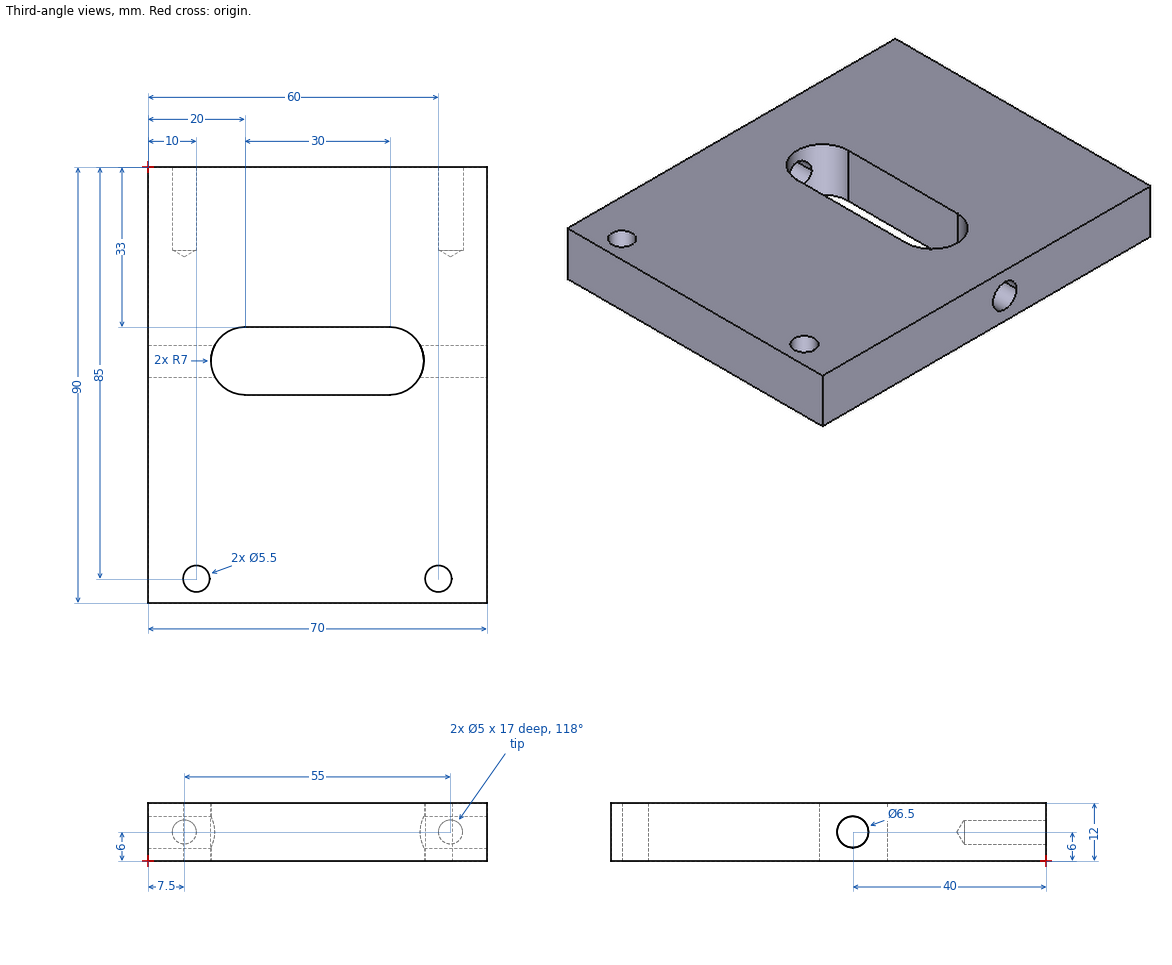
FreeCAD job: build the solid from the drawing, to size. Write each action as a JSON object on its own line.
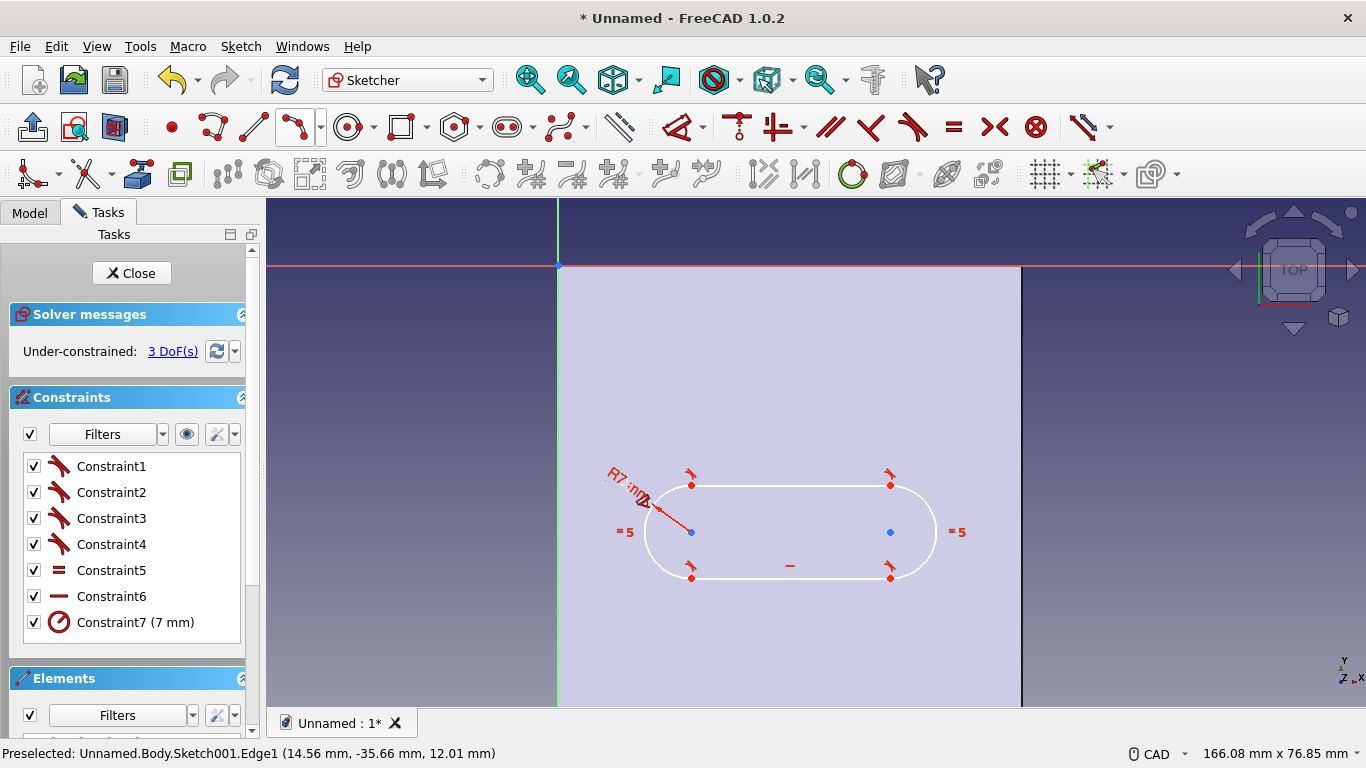
{"action": "left_click", "coordinate": [751, 486]}
{"action": "left_click", "coordinate": [791, 520]}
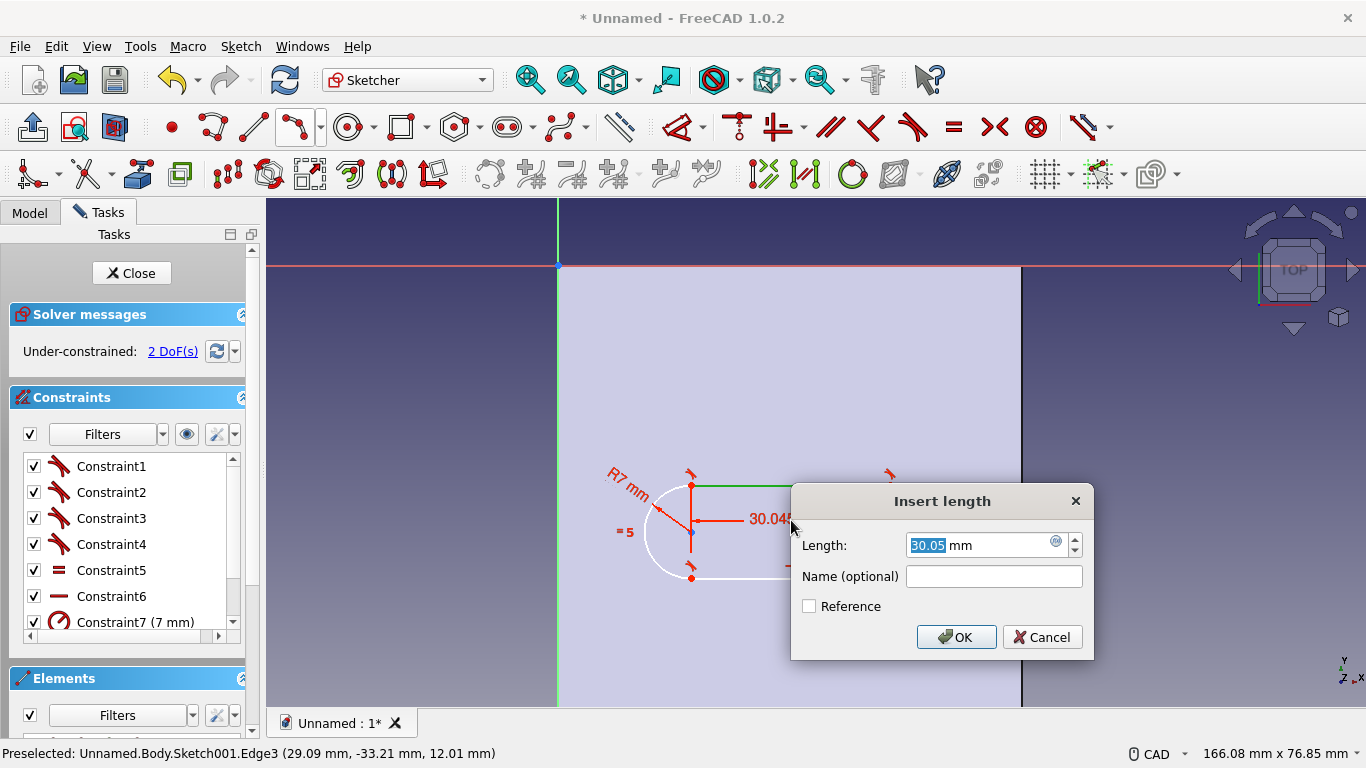
{"action": "type", "text": "30"}
{"action": "key", "text": "Return"}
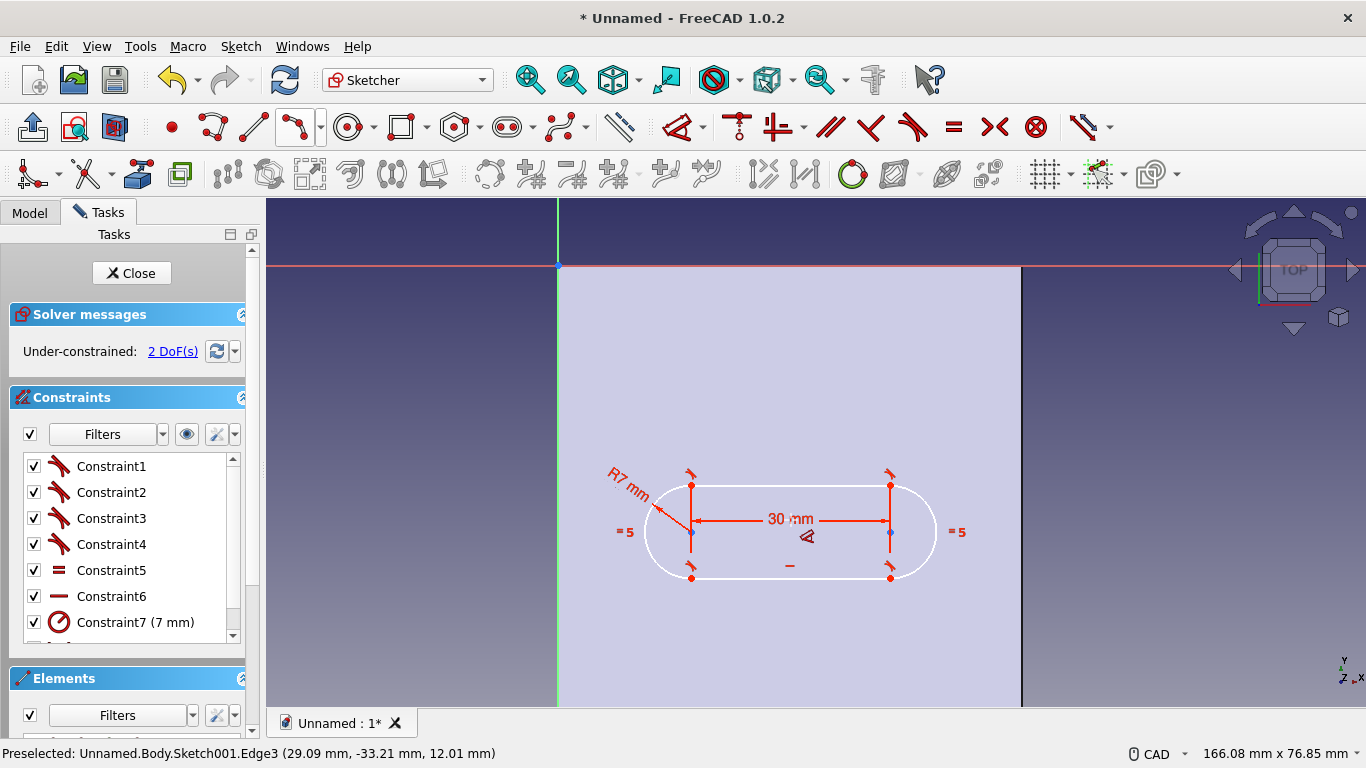
{"action": "left_click", "coordinate": [691, 486]}
{"action": "left_click", "coordinate": [625, 232]}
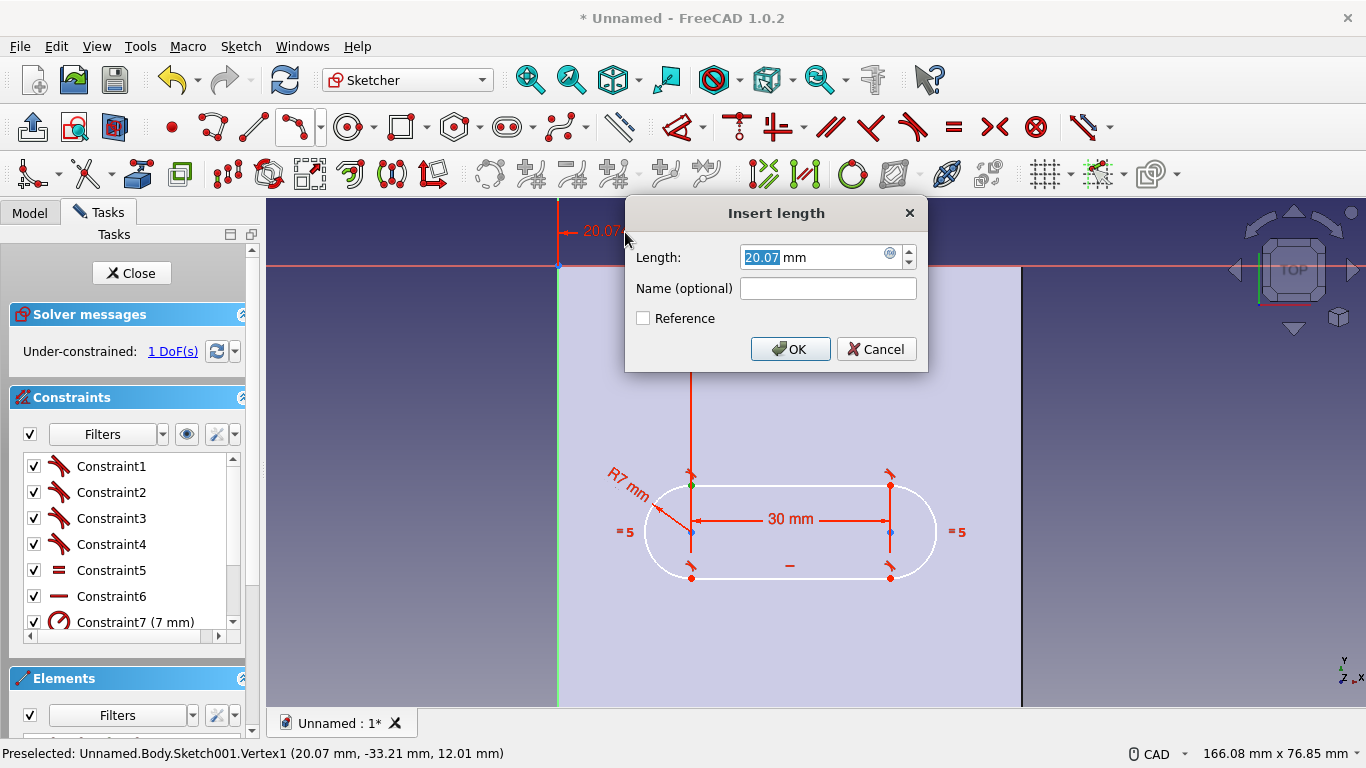
{"action": "type", "text": "20"}
{"action": "key", "text": "Return"}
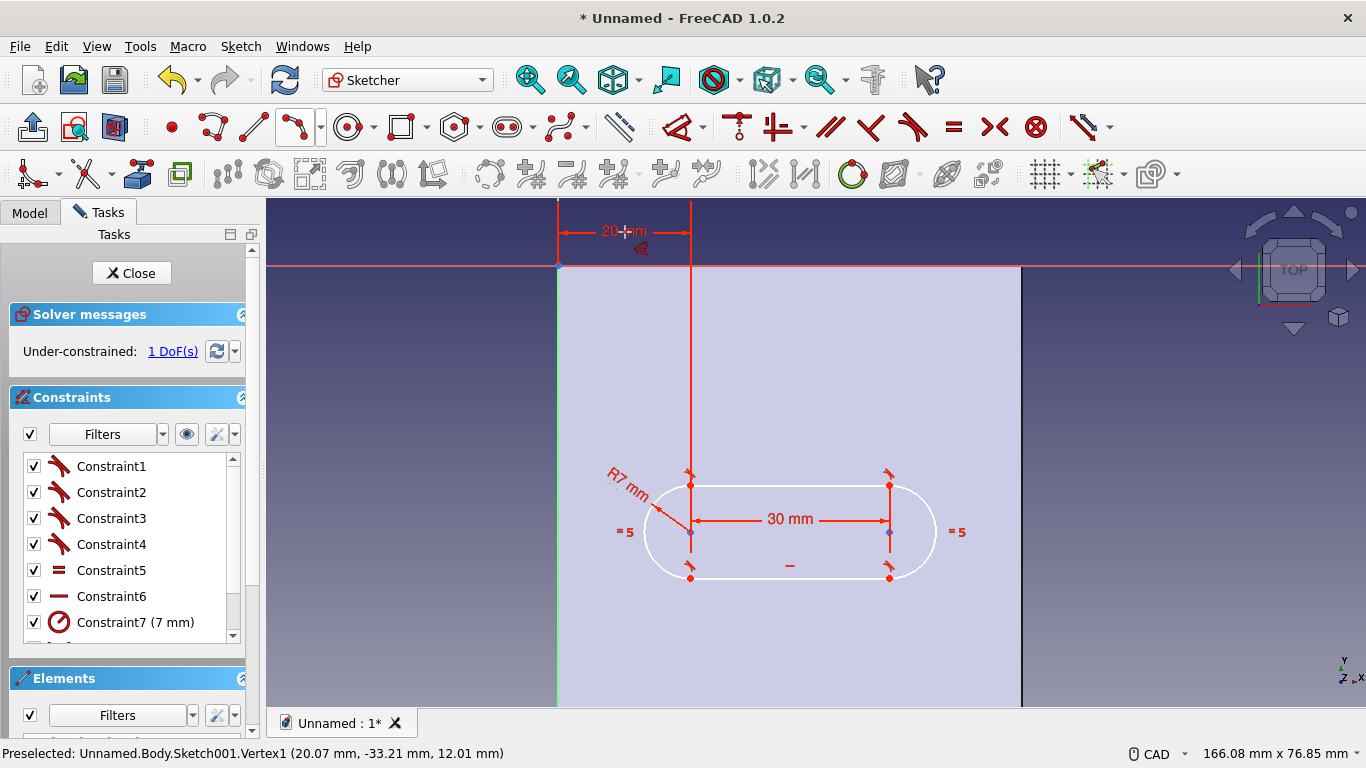
{"action": "left_click", "coordinate": [691, 486]}
{"action": "left_click", "coordinate": [524, 376]}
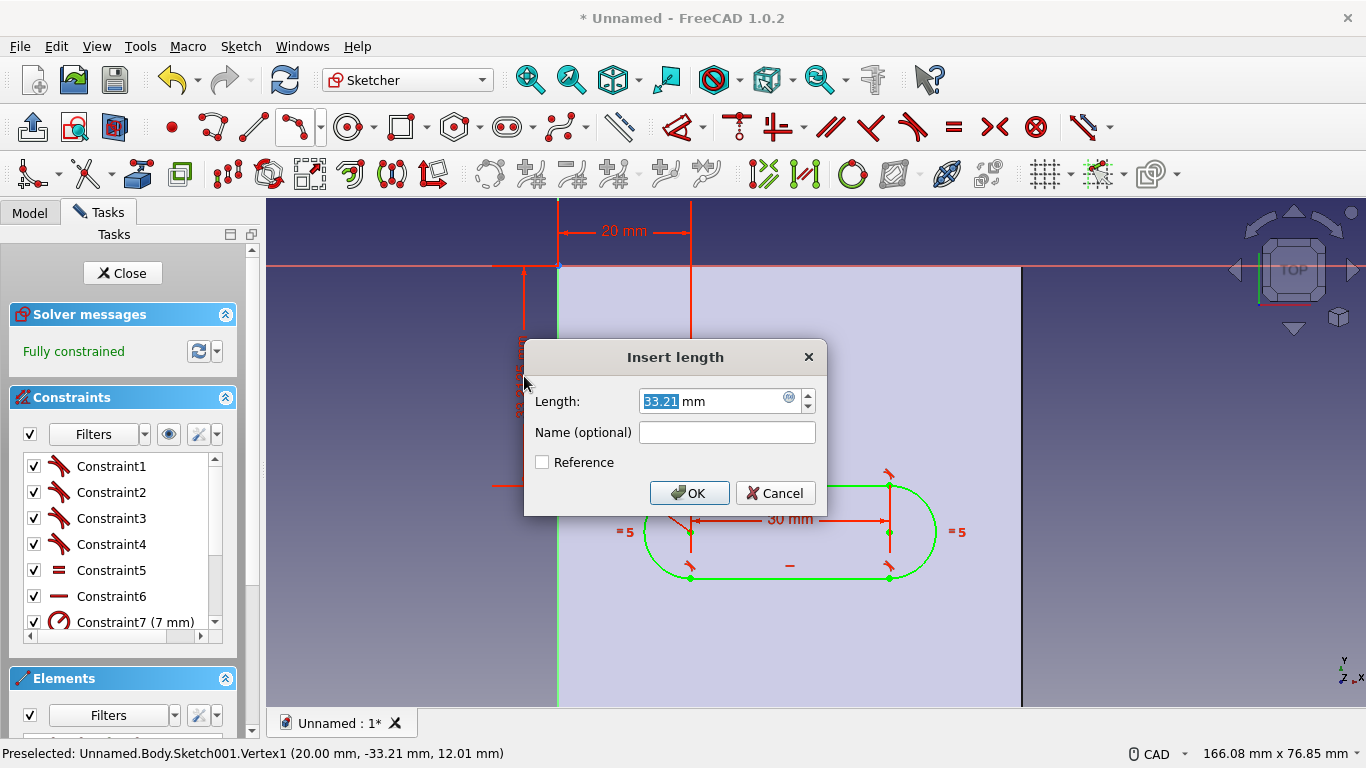
{"action": "type", "text": "33"}
{"action": "key", "text": "Return"}
{"action": "key", "text": "Escape"}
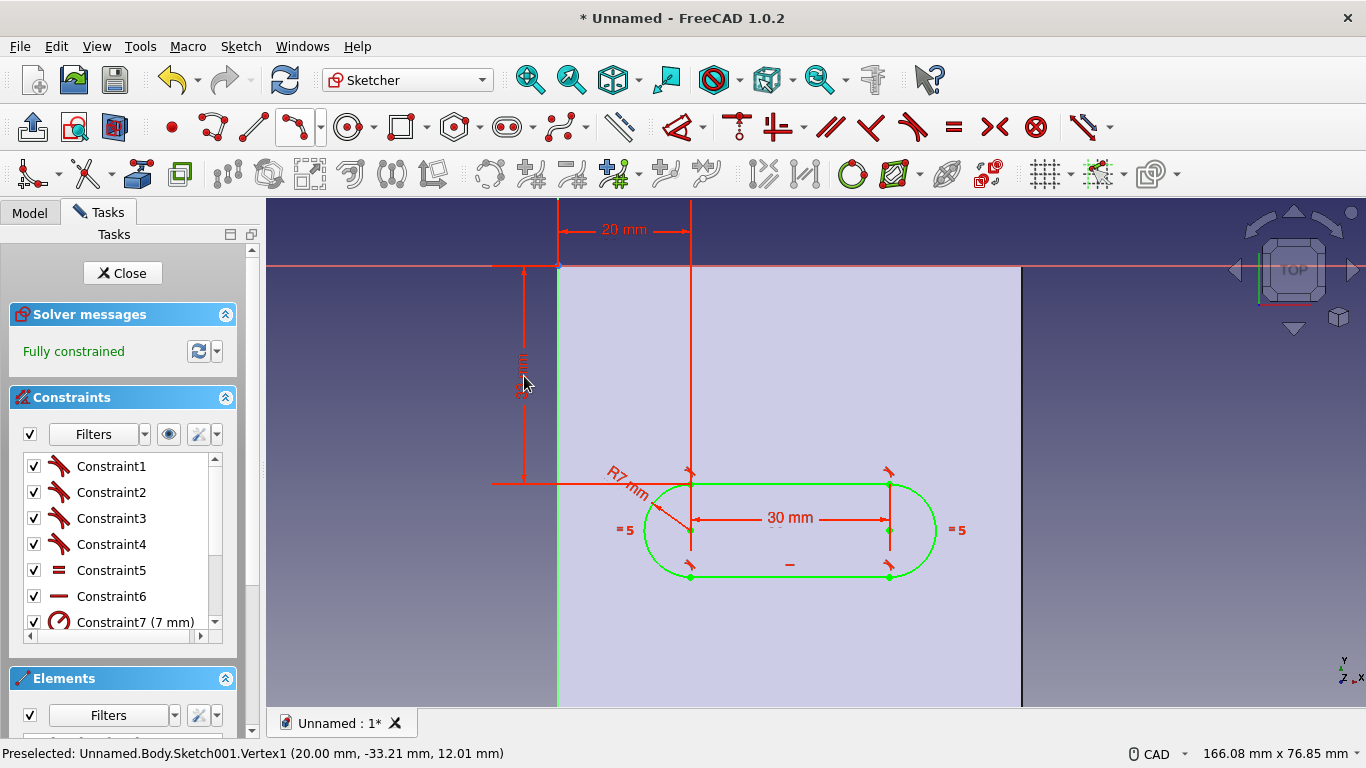
{"action": "left_click", "coordinate": [123, 273]}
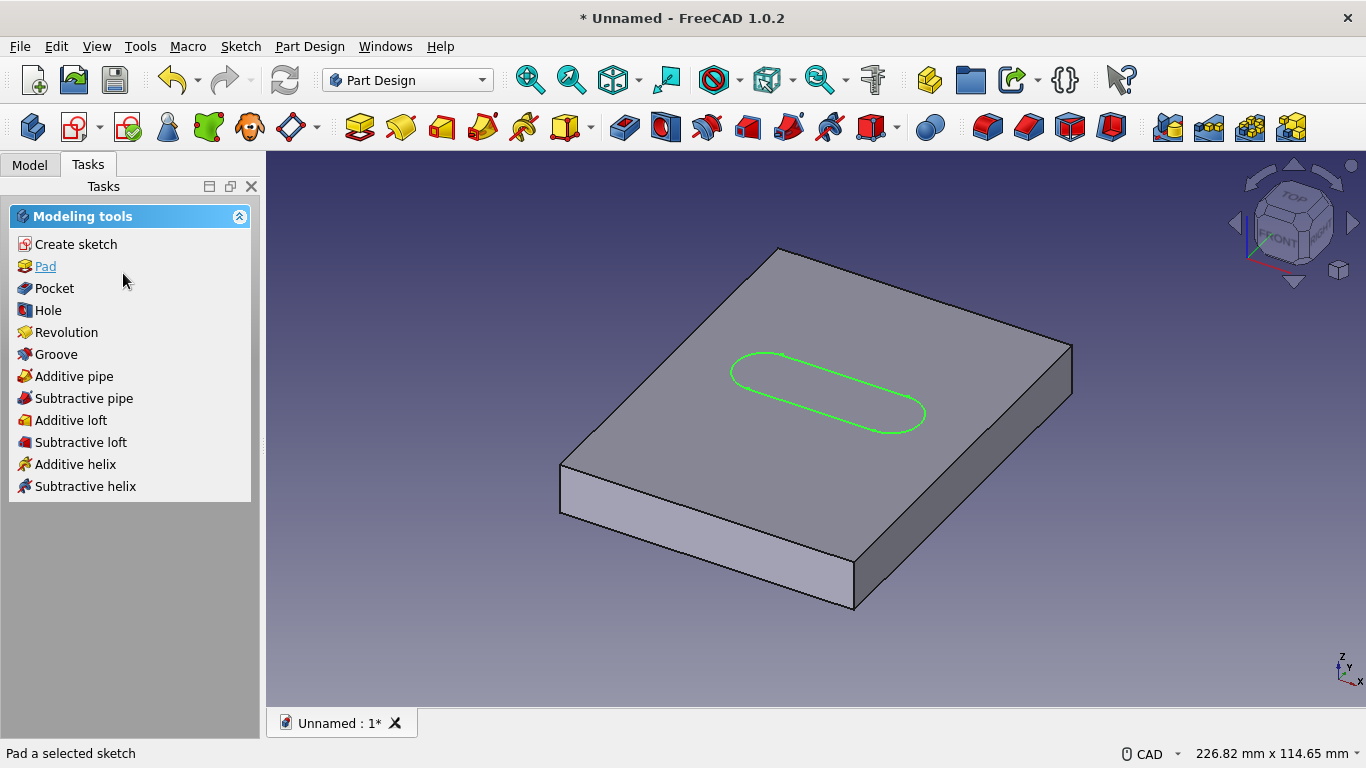
{"action": "left_click", "coordinate": [625, 128]}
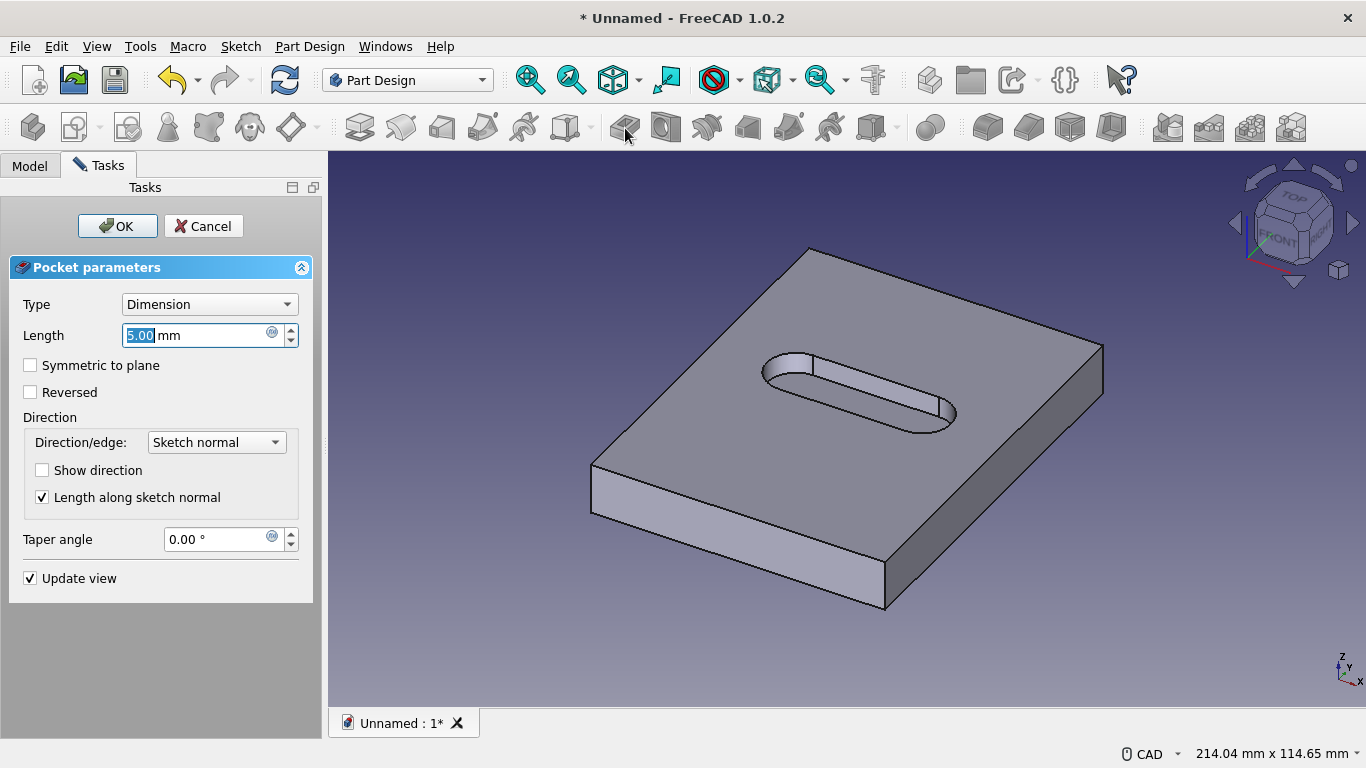
{"action": "left_click", "coordinate": [210, 304]}